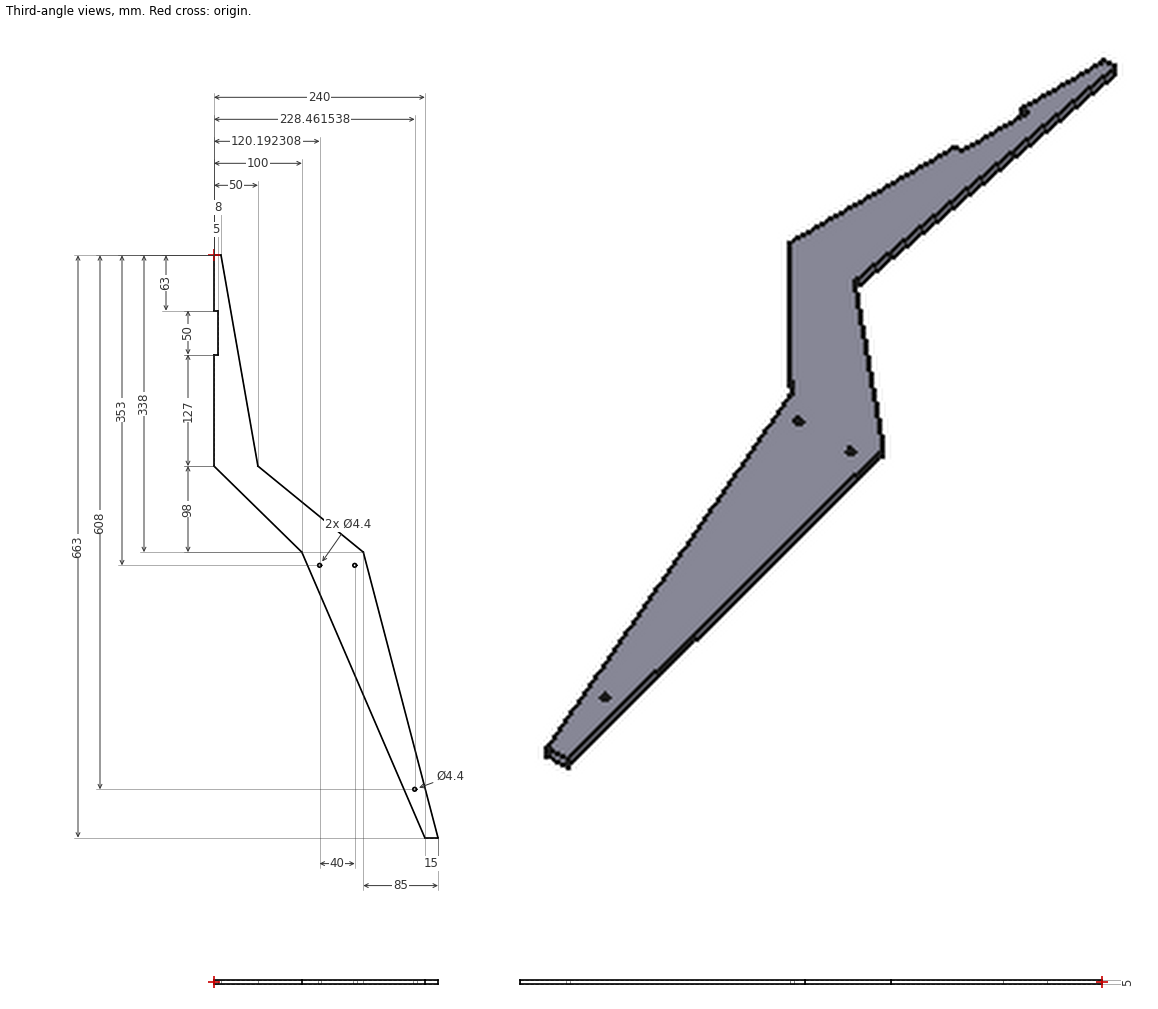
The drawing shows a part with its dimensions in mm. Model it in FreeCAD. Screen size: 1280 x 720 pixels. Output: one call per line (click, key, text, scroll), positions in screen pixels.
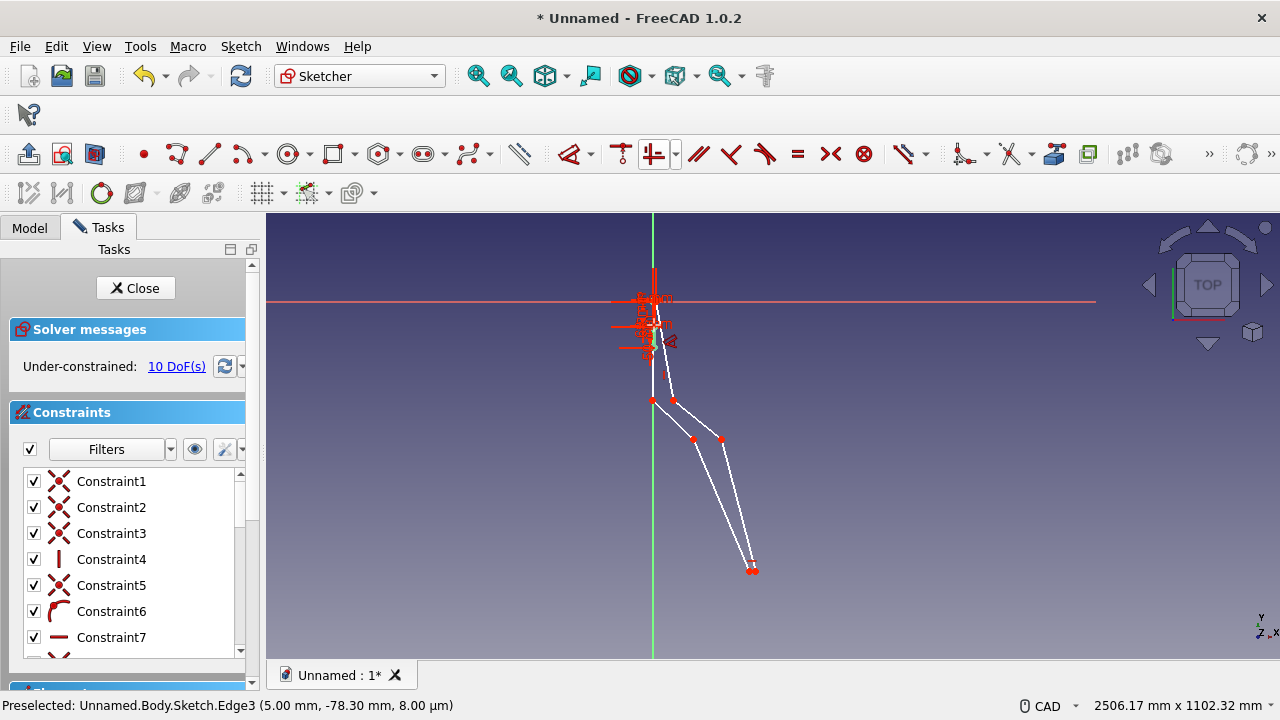
scroll(751, 571, up, 10)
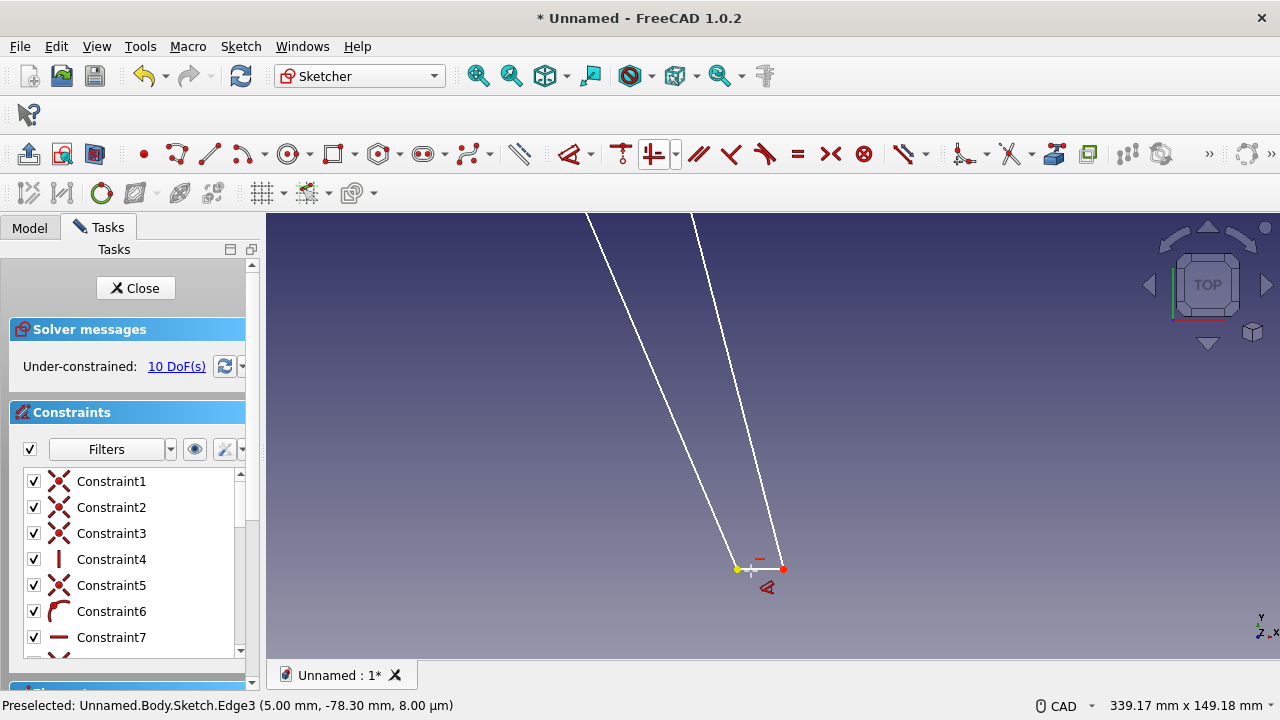
click(751, 569)
click(761, 603)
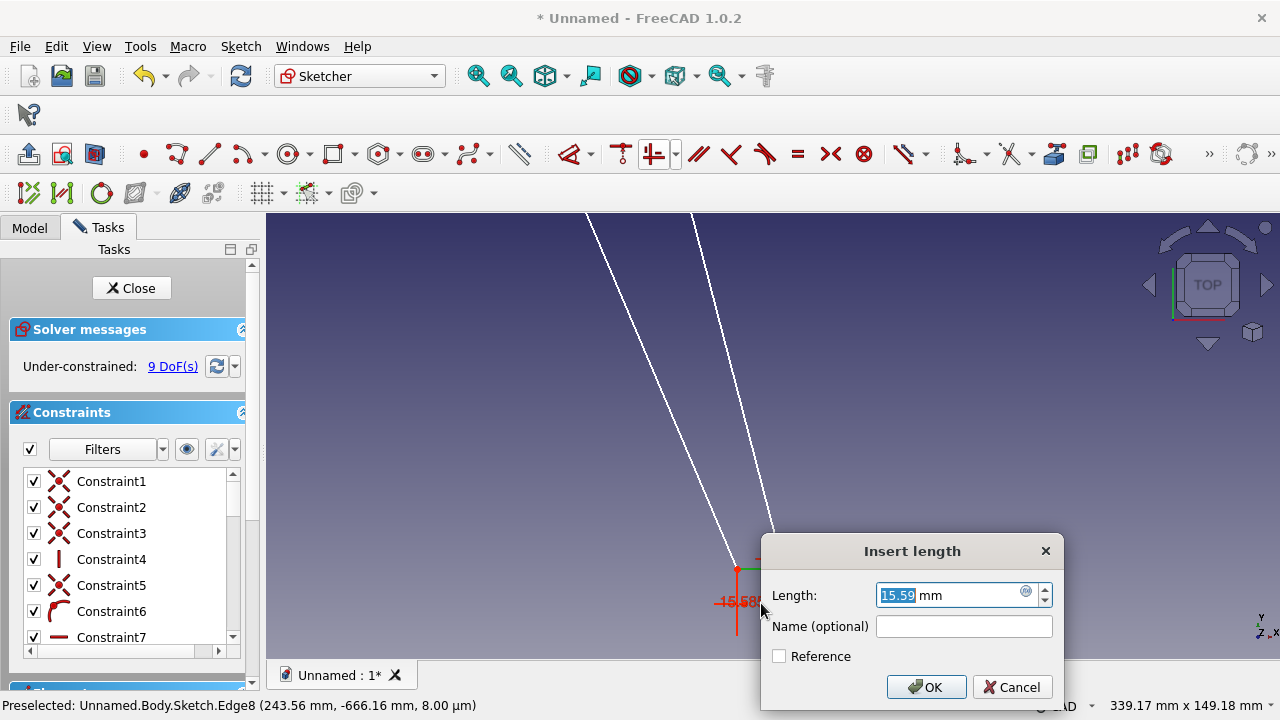
text(15)
key(Return)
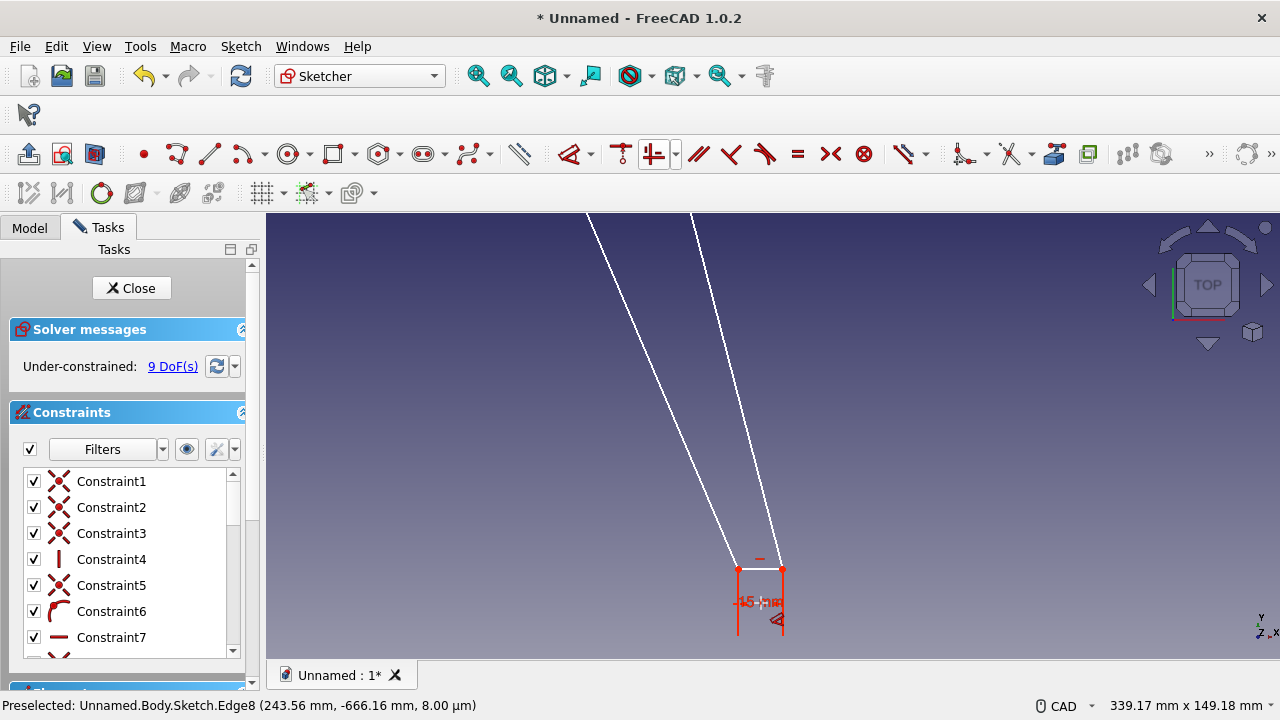
scroll(752, 572, down, 10)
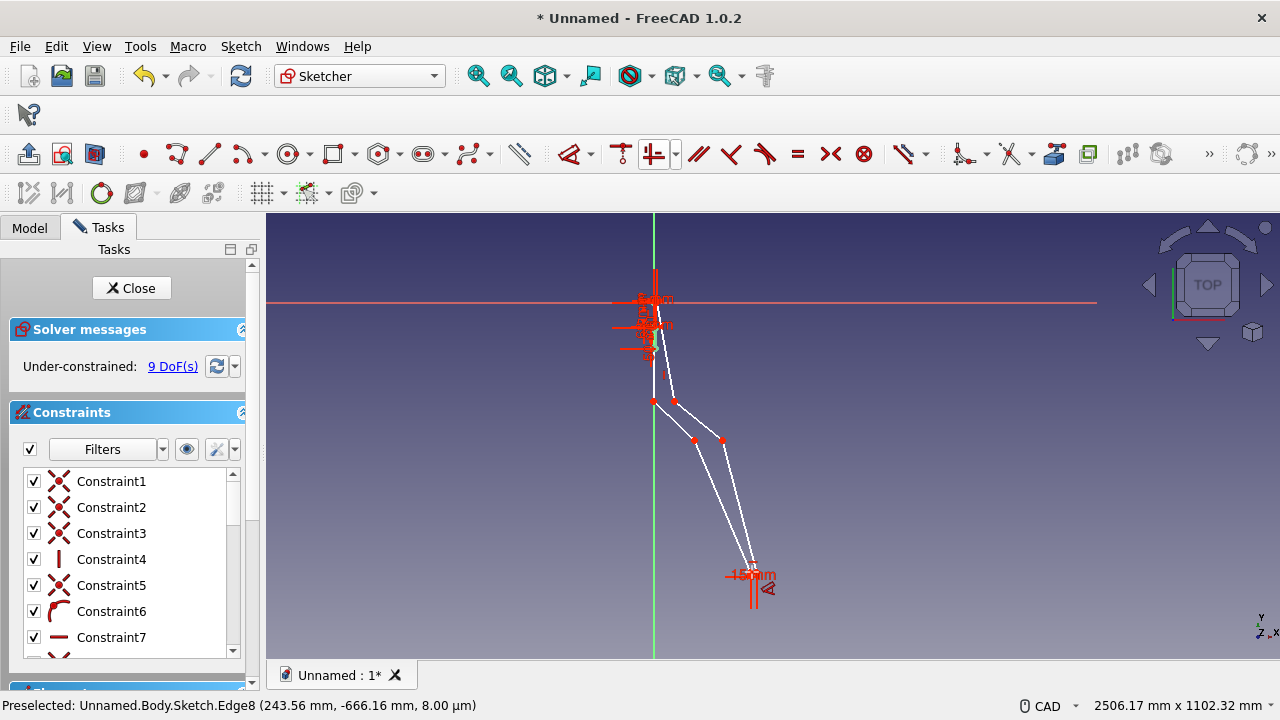
click(654, 364)
click(620, 375)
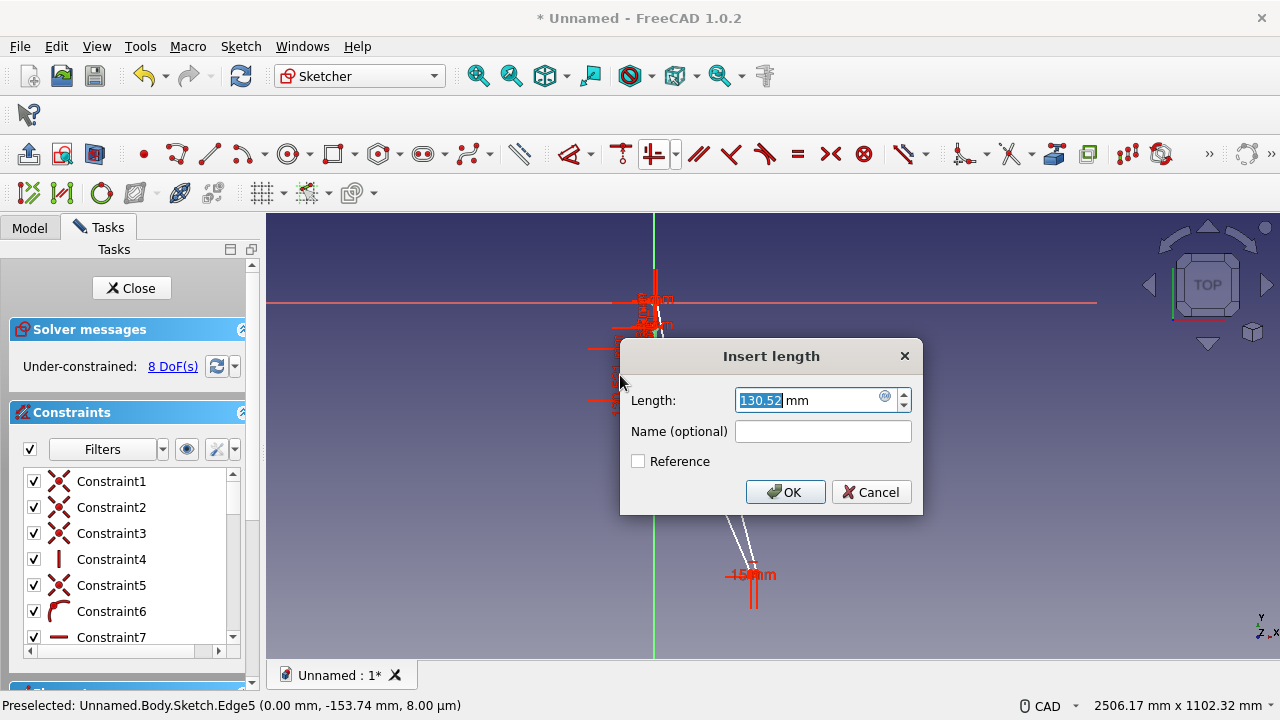
text(127)
key(Return)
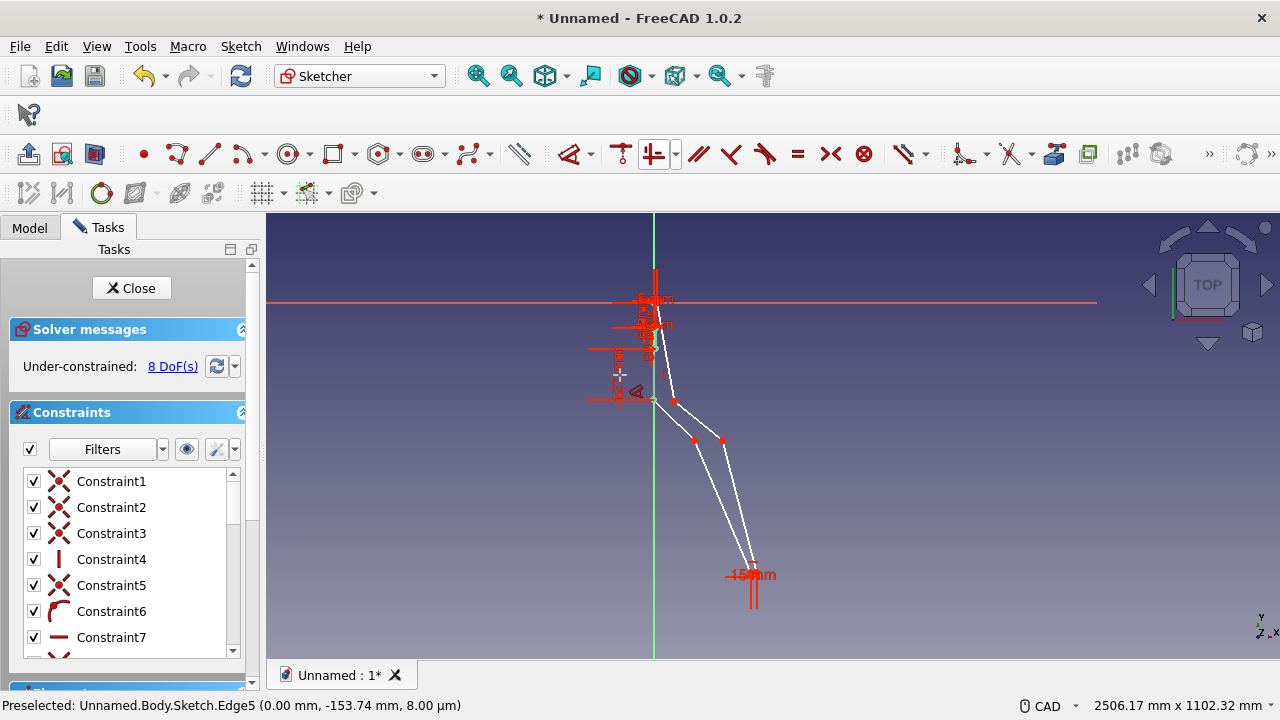
scroll(674, 401, up, 4)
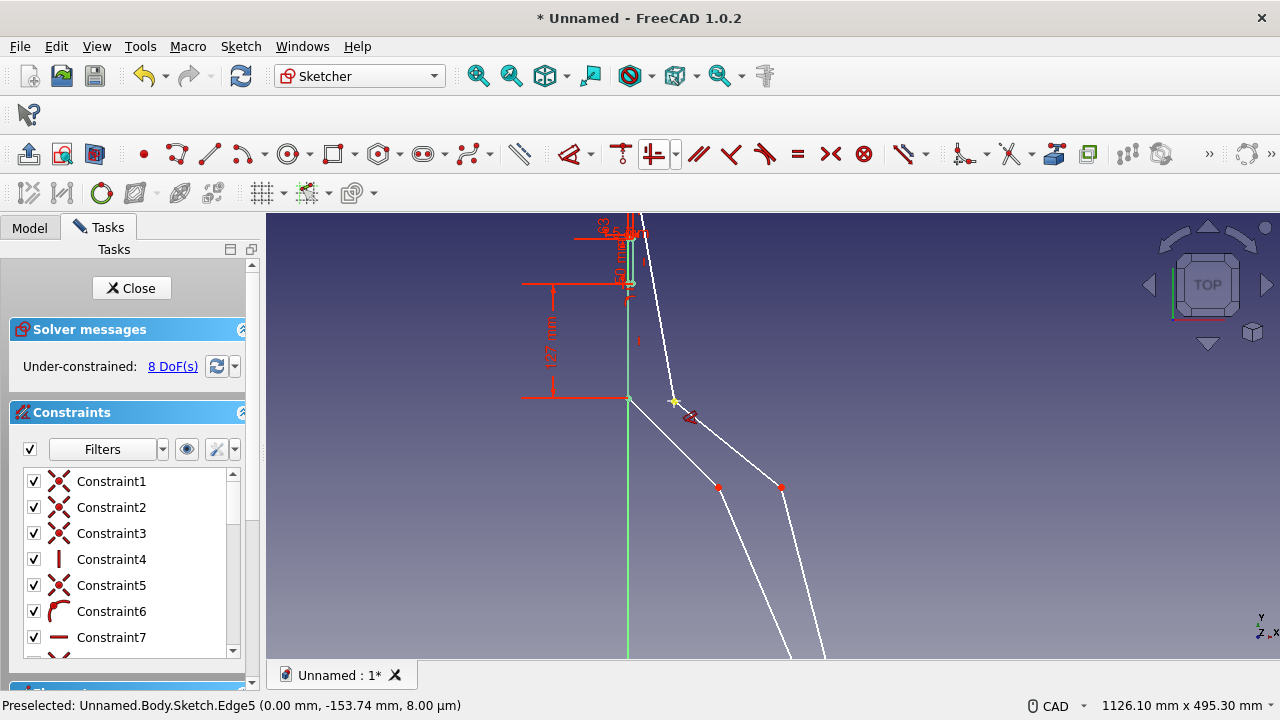
click(674, 401)
click(651, 459)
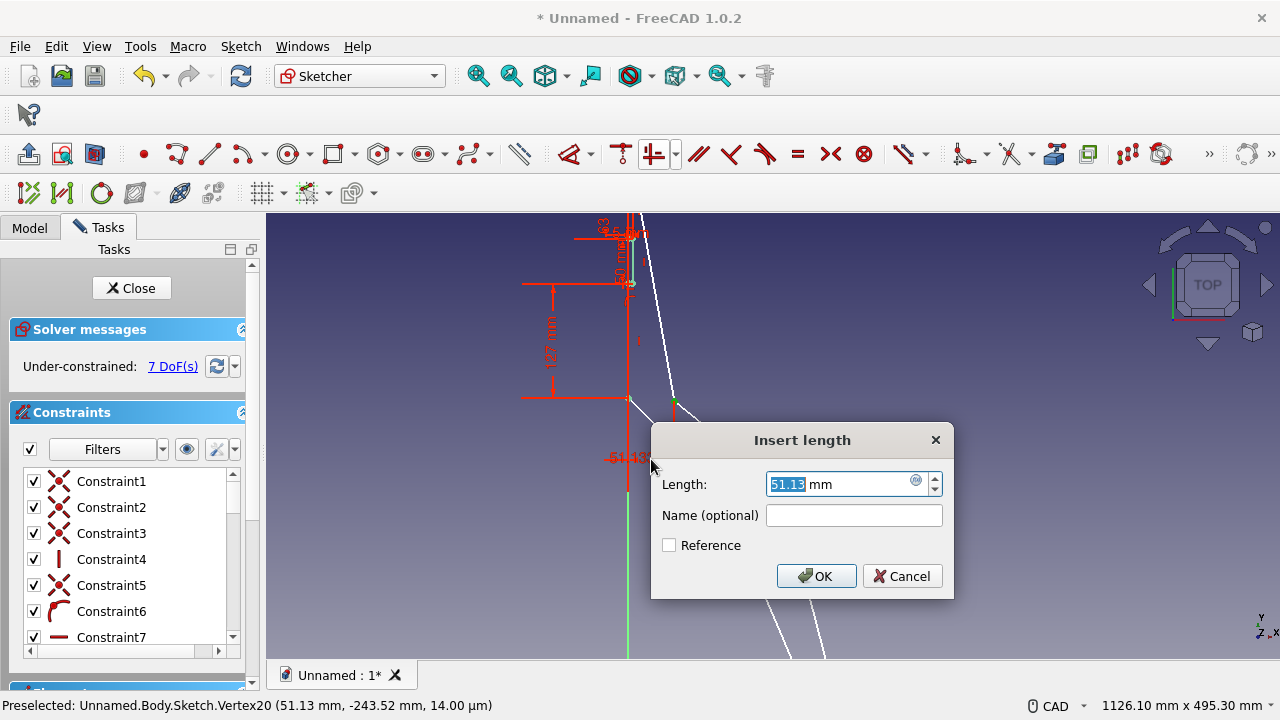
text(50)
key(Return)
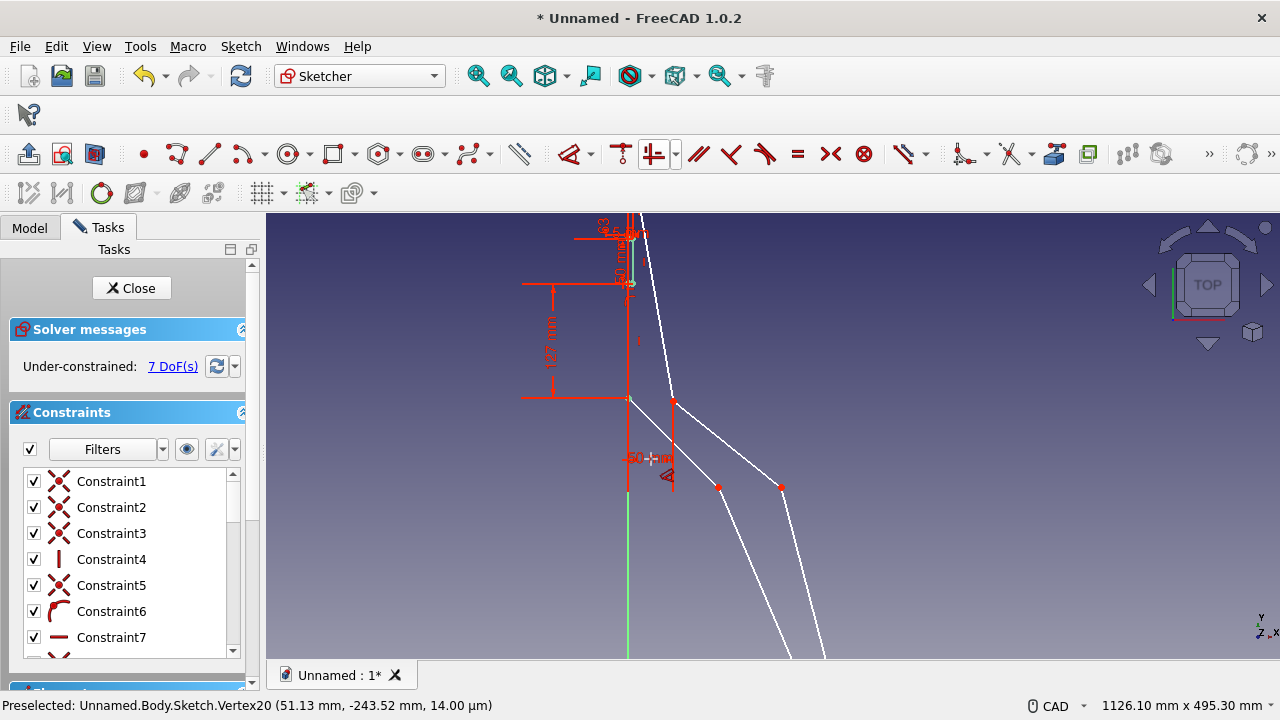
click(656, 425)
click(594, 422)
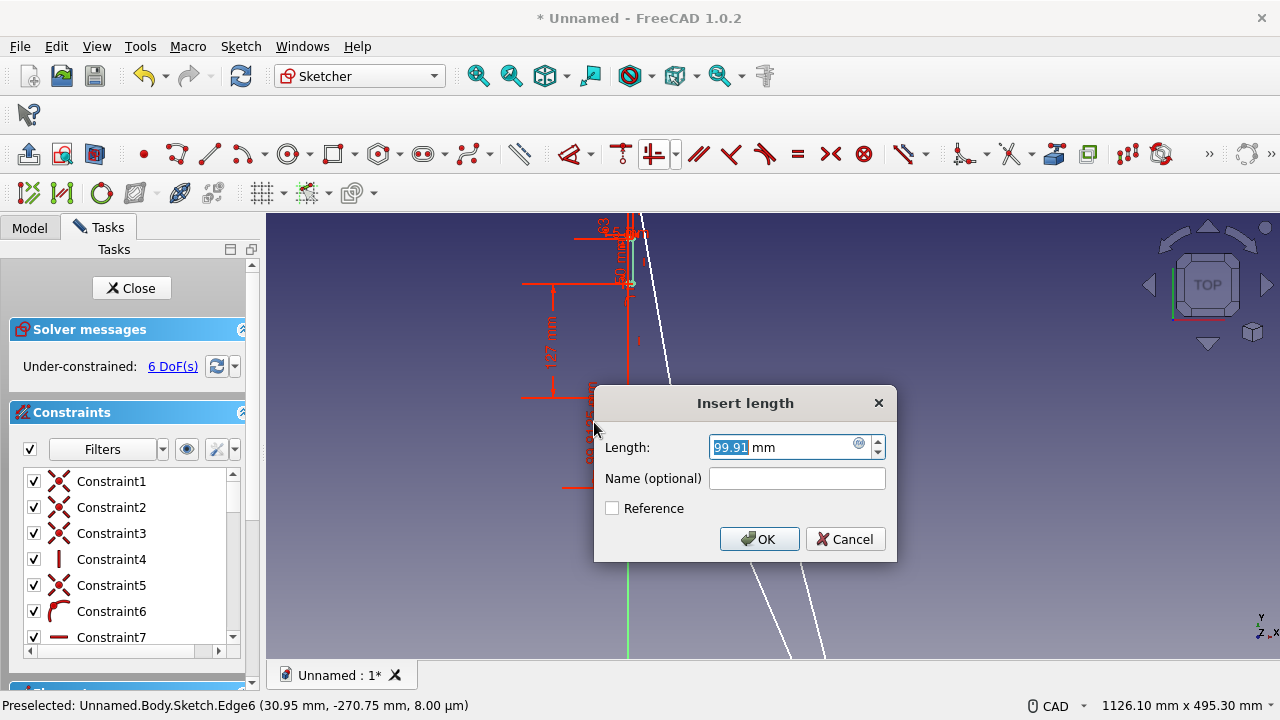
text(98)
key(Return)